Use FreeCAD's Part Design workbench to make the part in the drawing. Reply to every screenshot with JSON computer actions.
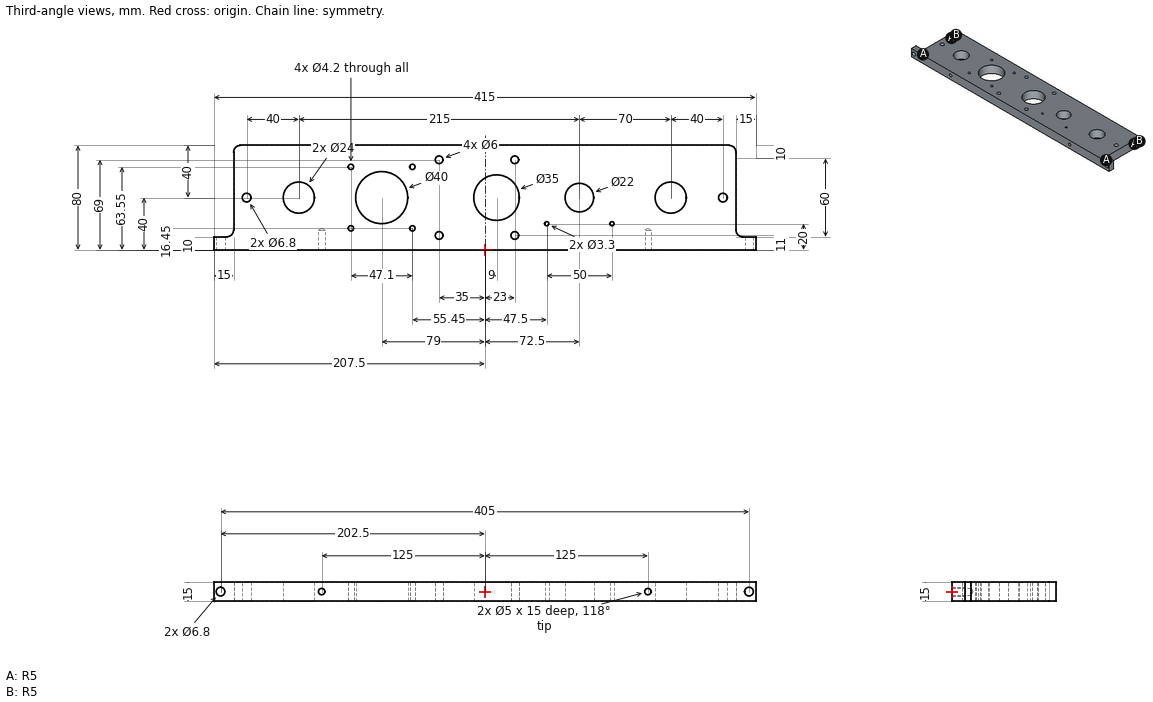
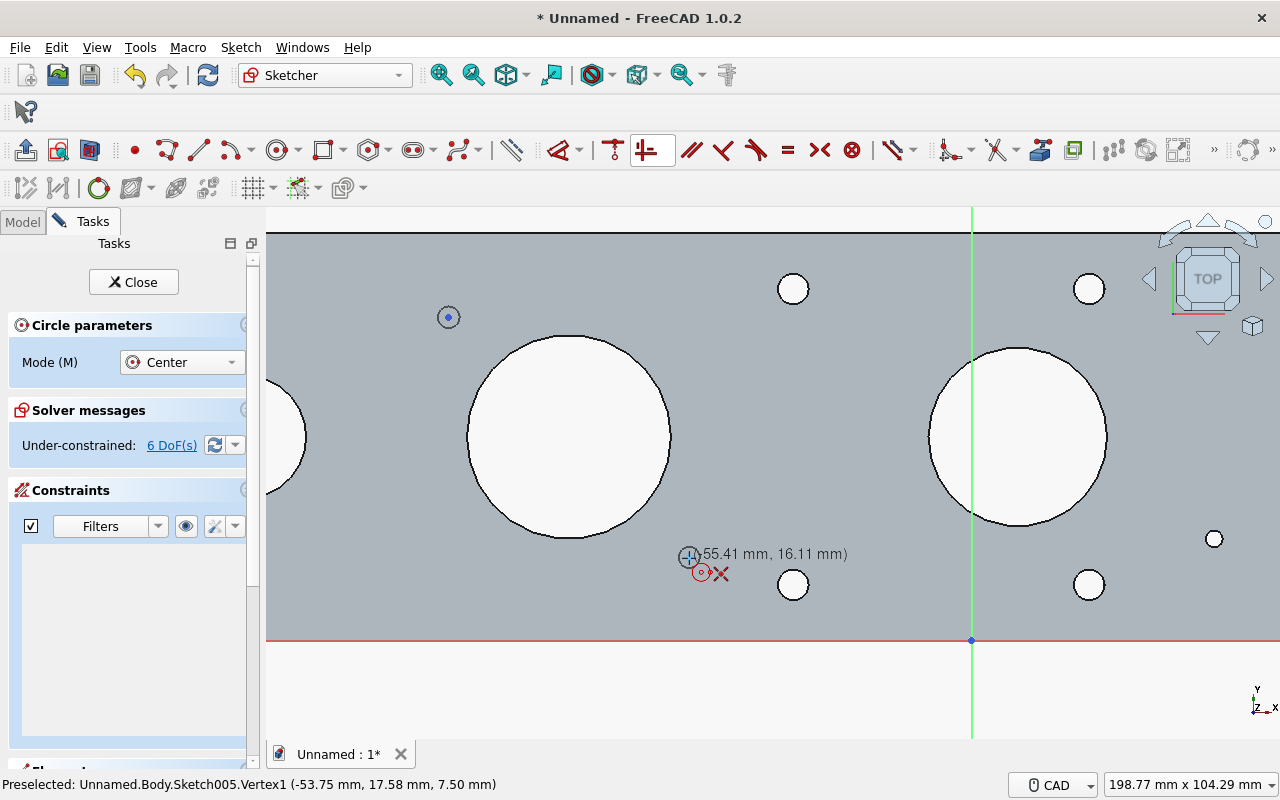
{"action": "scroll", "coordinate": [449, 557], "scroll_direction": "up", "scroll_amount": 4}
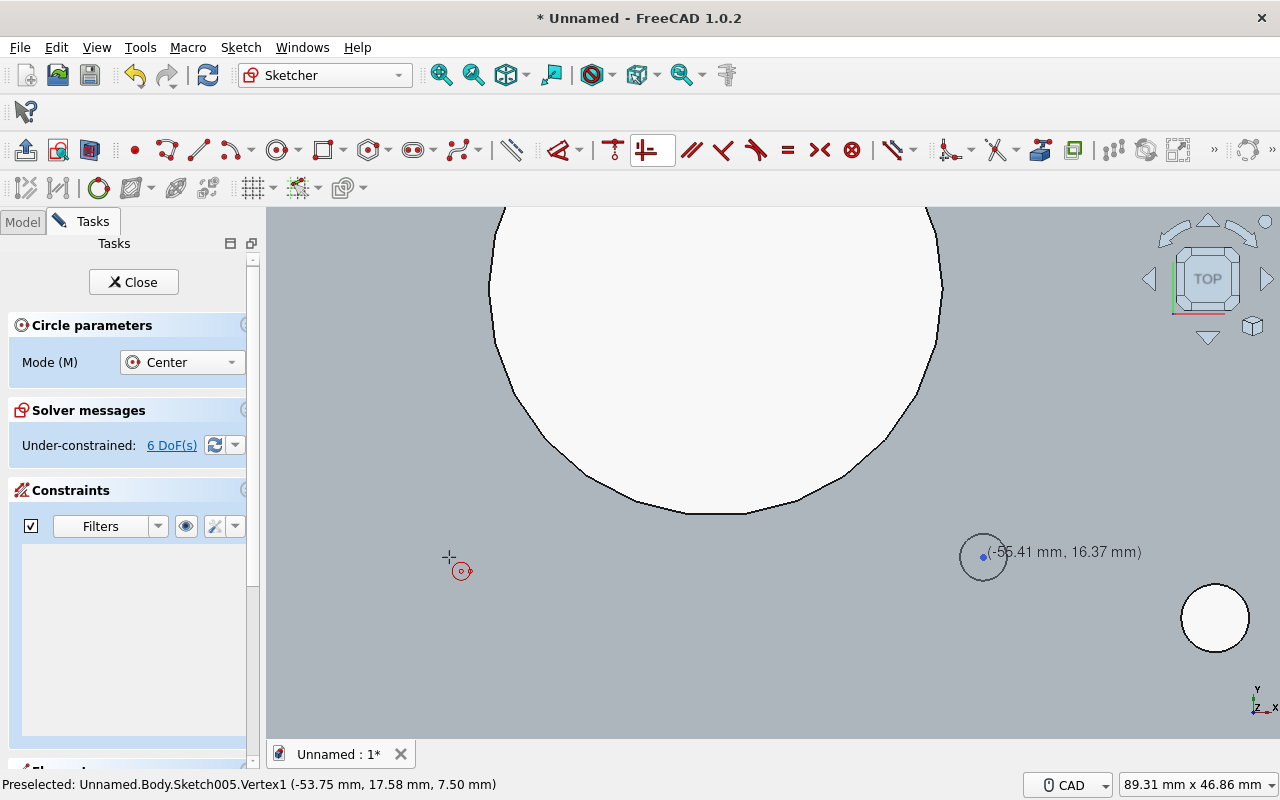
{"action": "left_click", "coordinate": [448, 556]}
{"action": "left_click", "coordinate": [465, 540]}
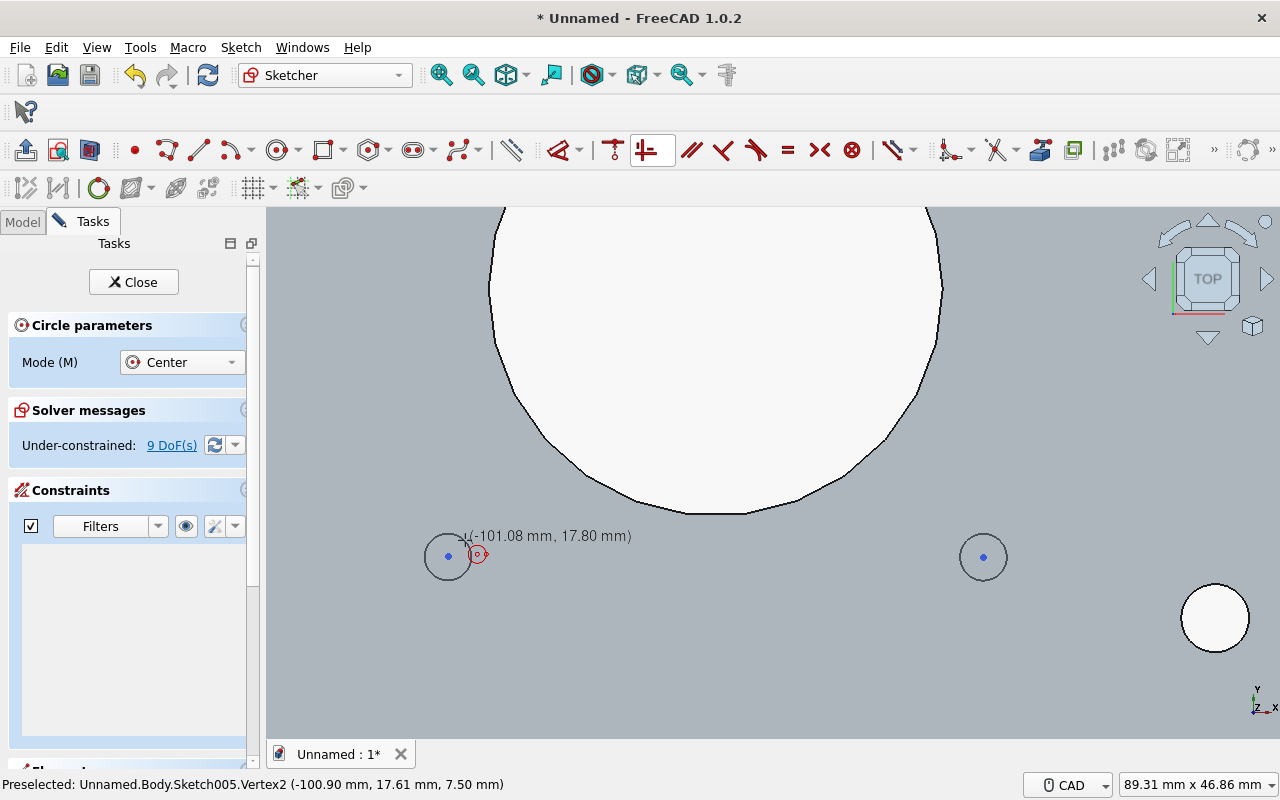
{"action": "scroll", "coordinate": [448, 557], "scroll_direction": "down", "scroll_amount": 4}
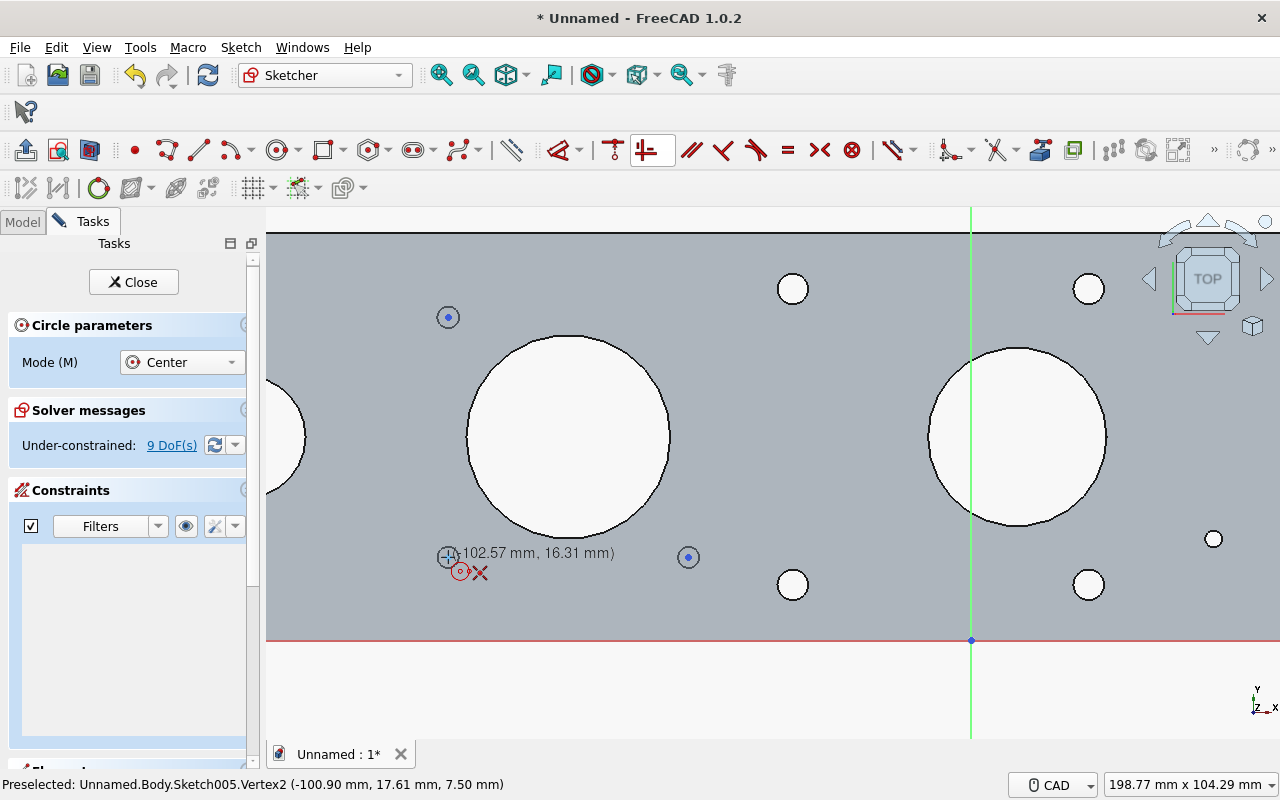
{"action": "scroll", "coordinate": [688, 317], "scroll_direction": "up", "scroll_amount": 4}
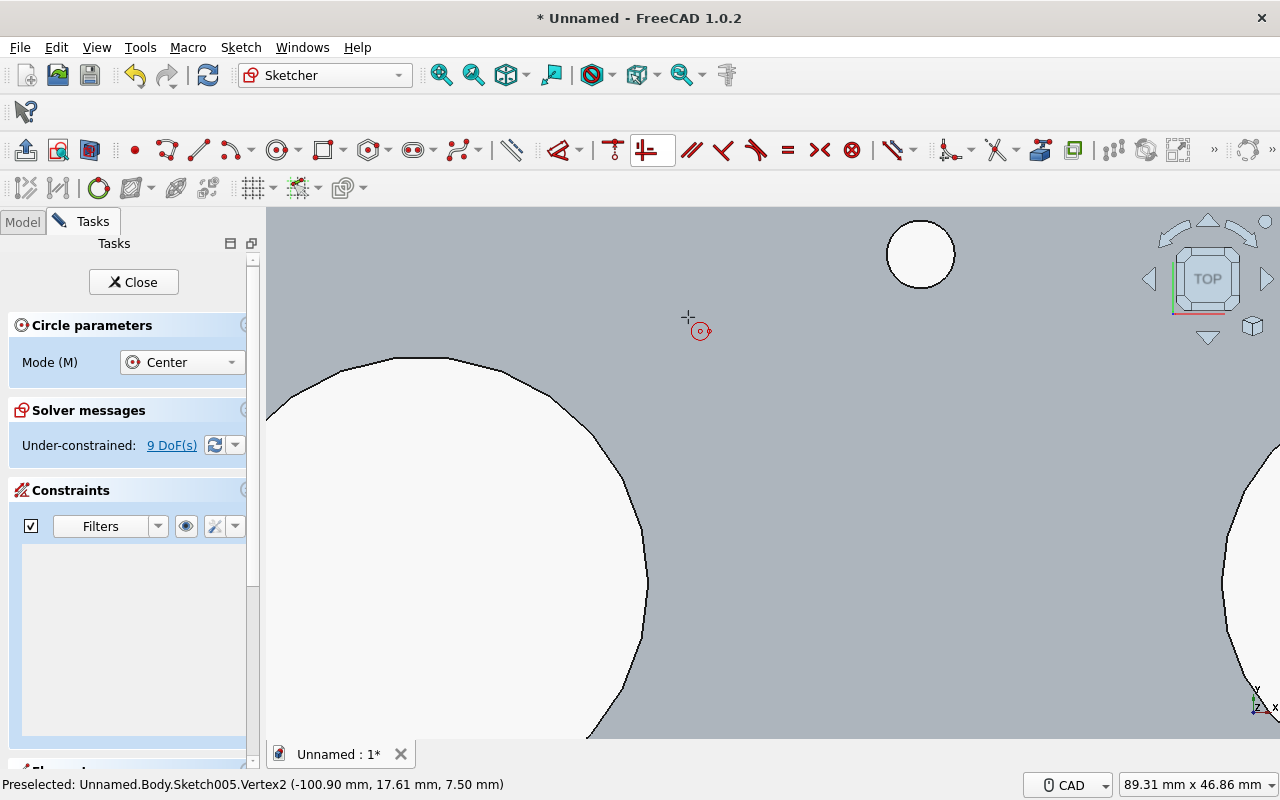
{"action": "left_click", "coordinate": [689, 316]}
{"action": "left_click", "coordinate": [705, 299]}
{"action": "key", "text": "Escape"}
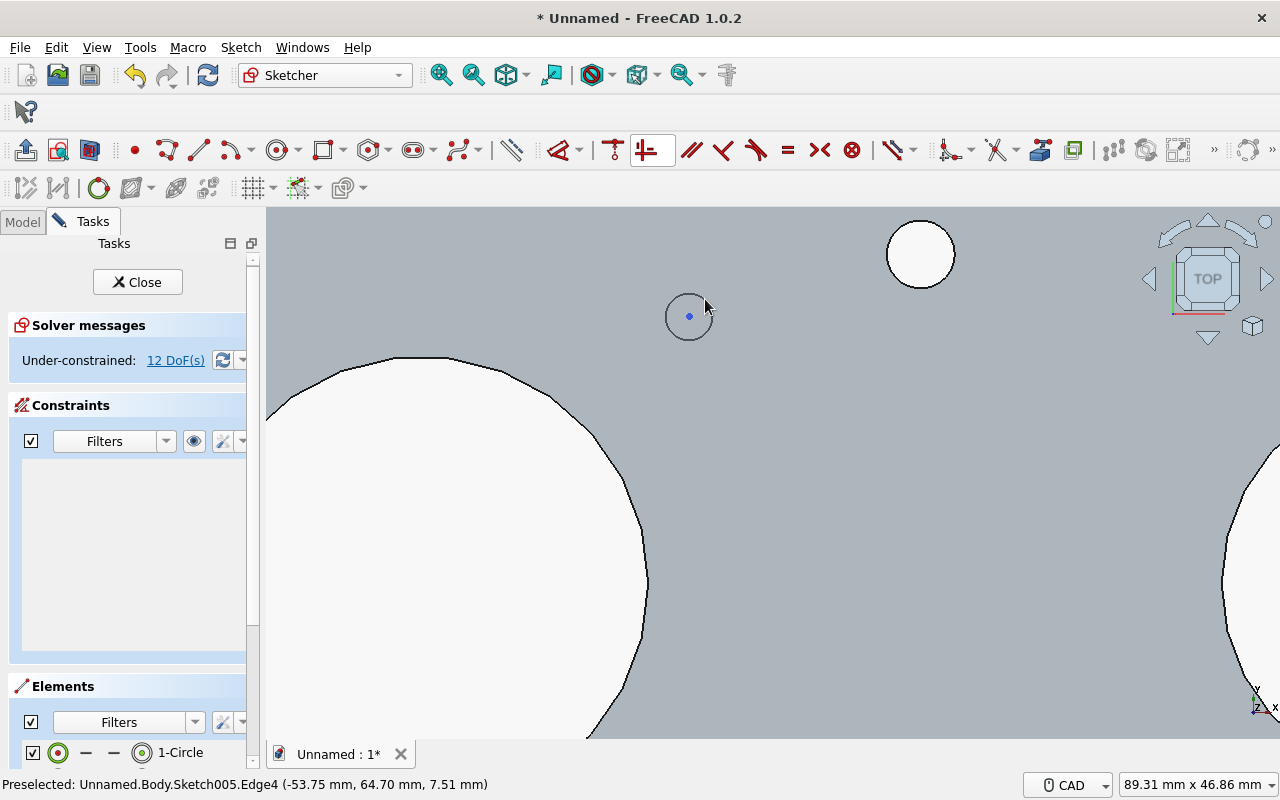
{"action": "scroll", "coordinate": [689, 316], "scroll_direction": "down", "scroll_amount": 4}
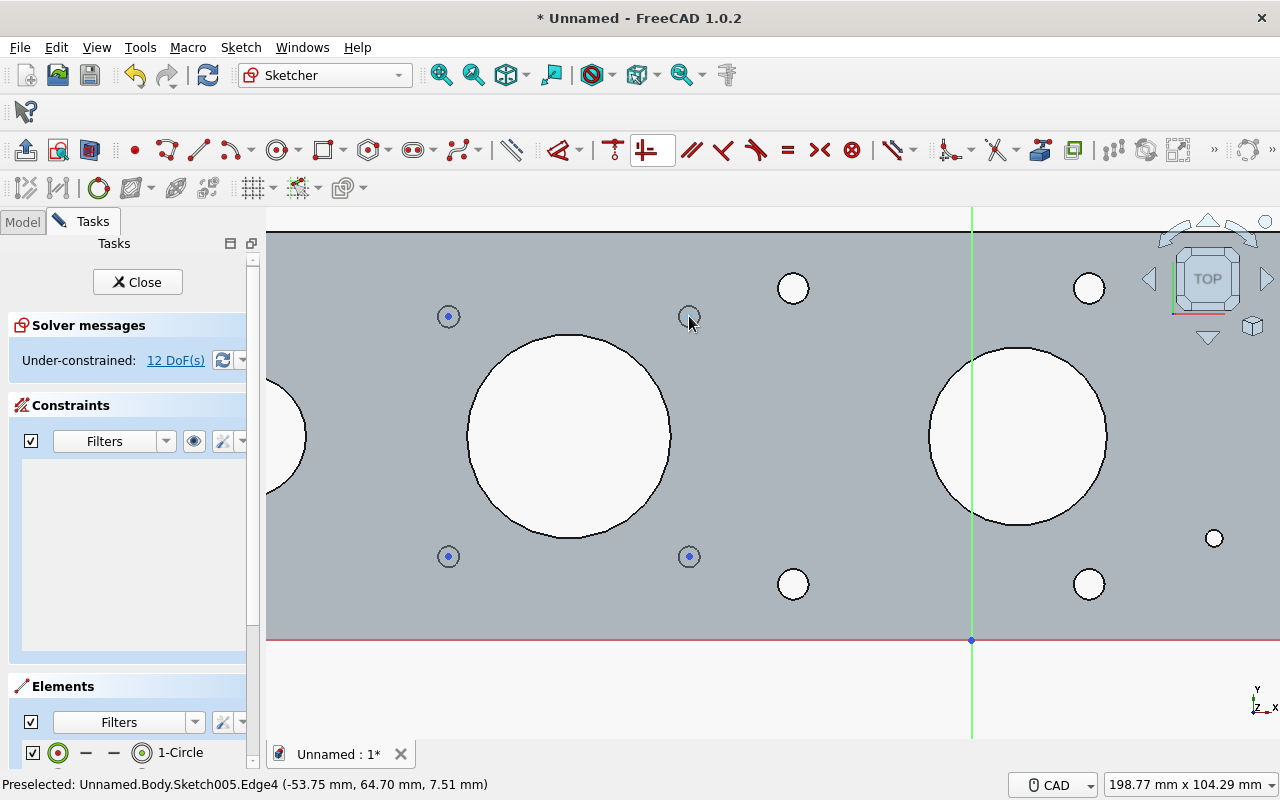
{"action": "scroll", "coordinate": [456, 309], "scroll_direction": "up", "scroll_amount": 2}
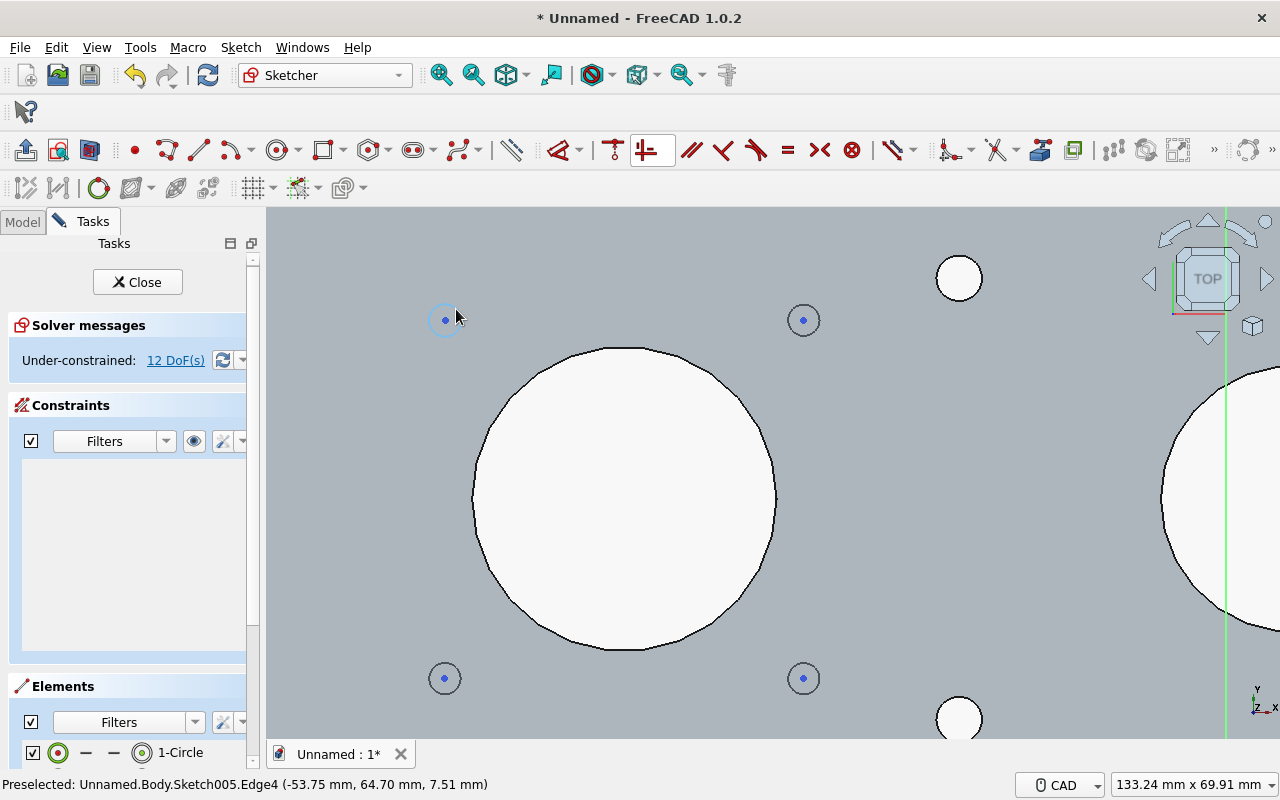
{"action": "left_click", "coordinate": [456, 309]}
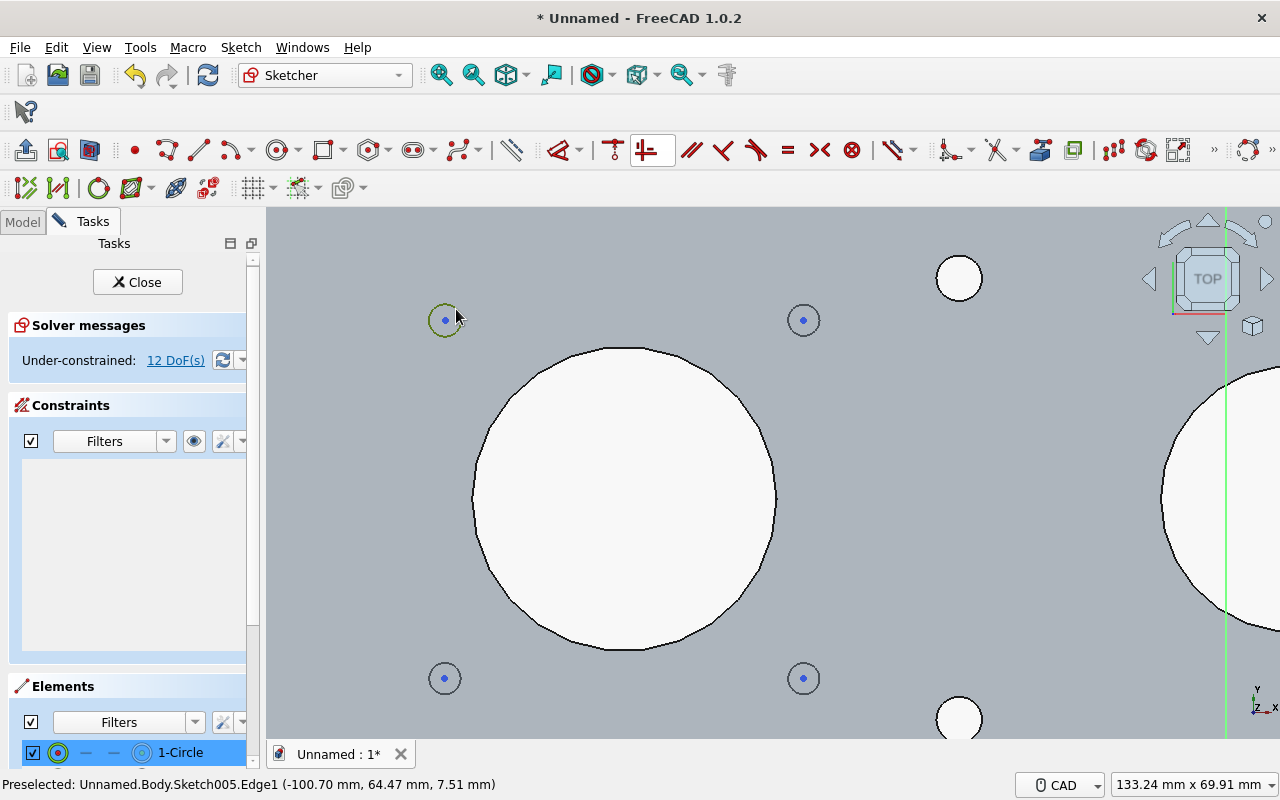
{"action": "left_click", "coordinate": [815, 668]}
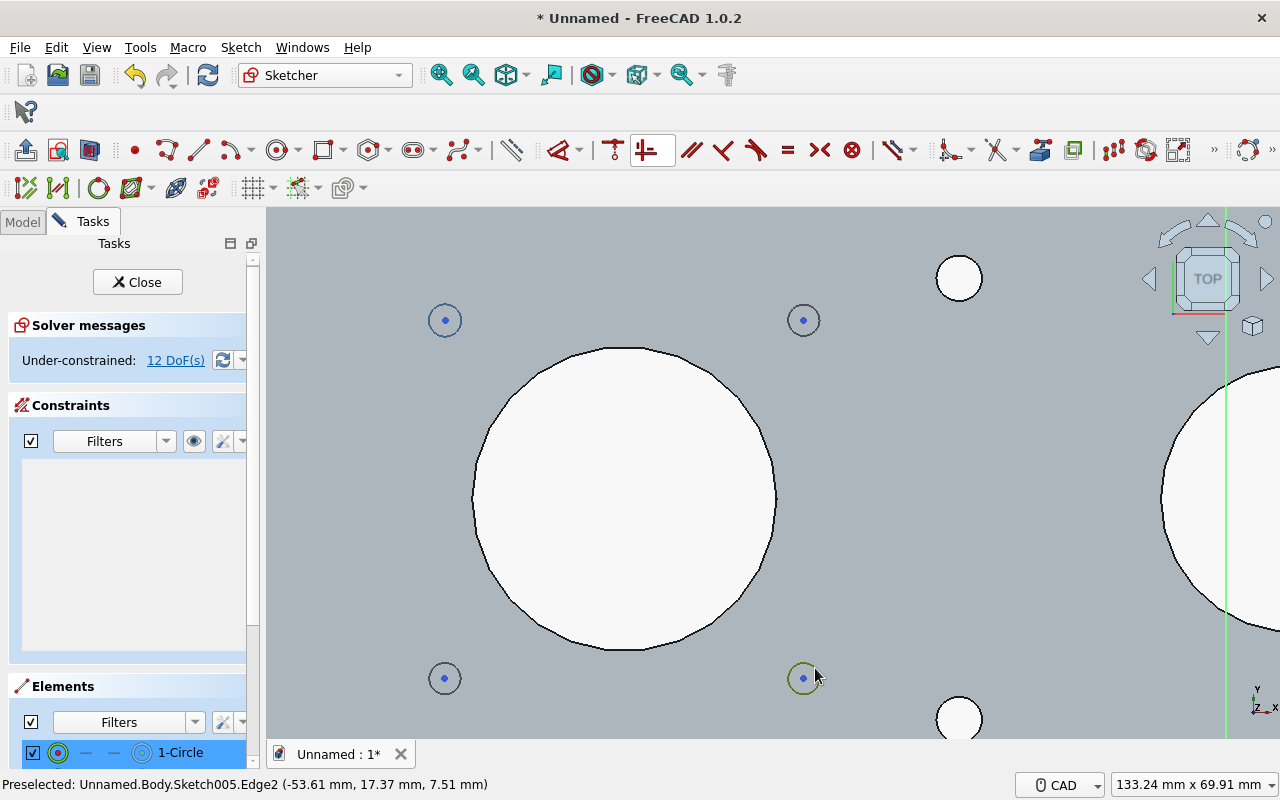
{"action": "left_click", "coordinate": [456, 667]}